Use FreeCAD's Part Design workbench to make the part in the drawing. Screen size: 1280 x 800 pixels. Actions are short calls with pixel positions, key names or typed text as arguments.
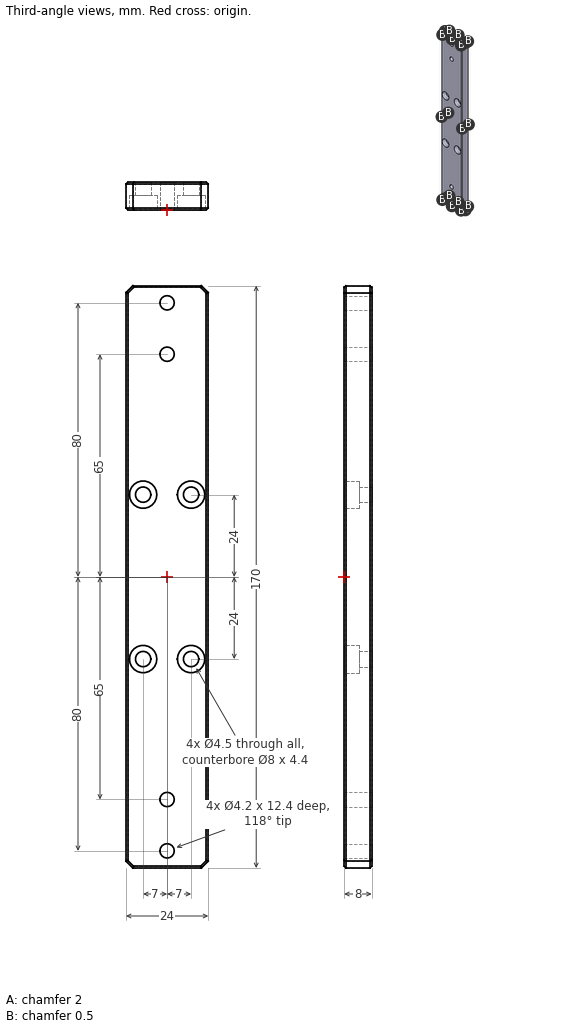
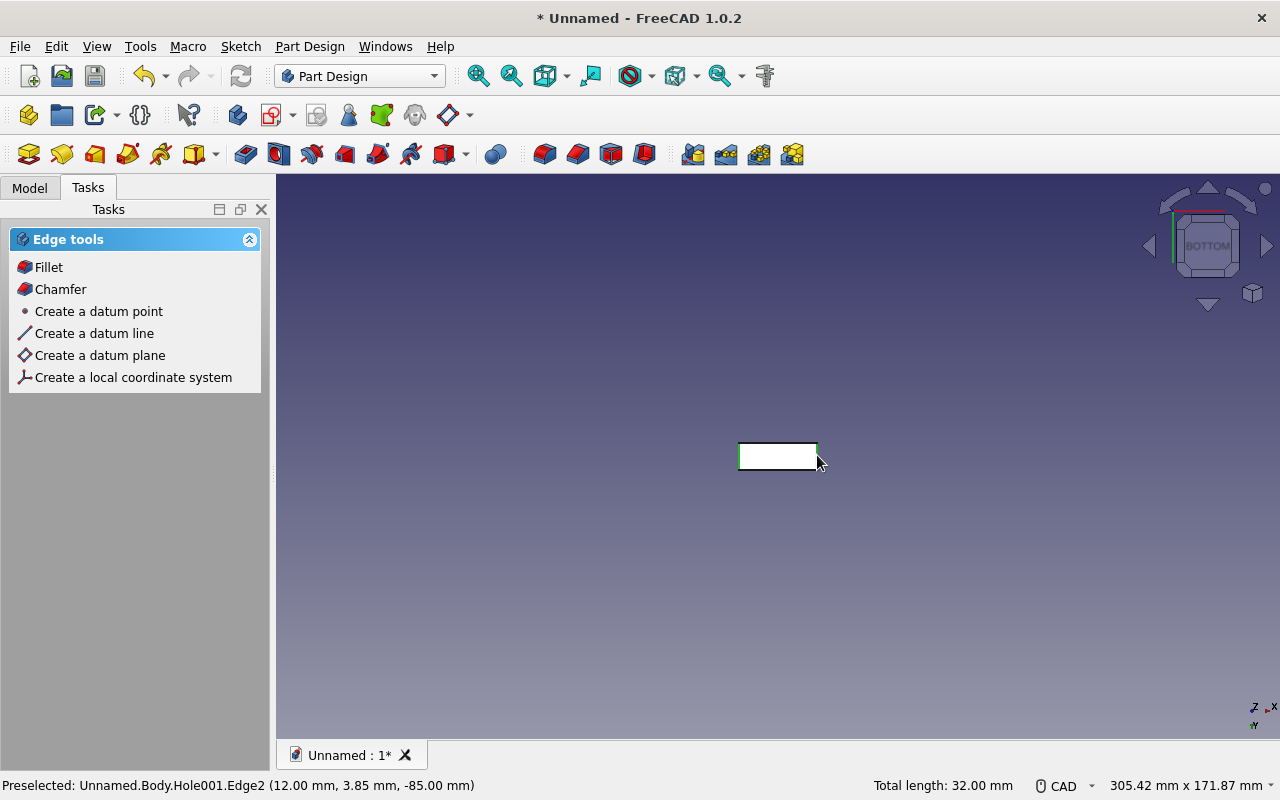
click(578, 154)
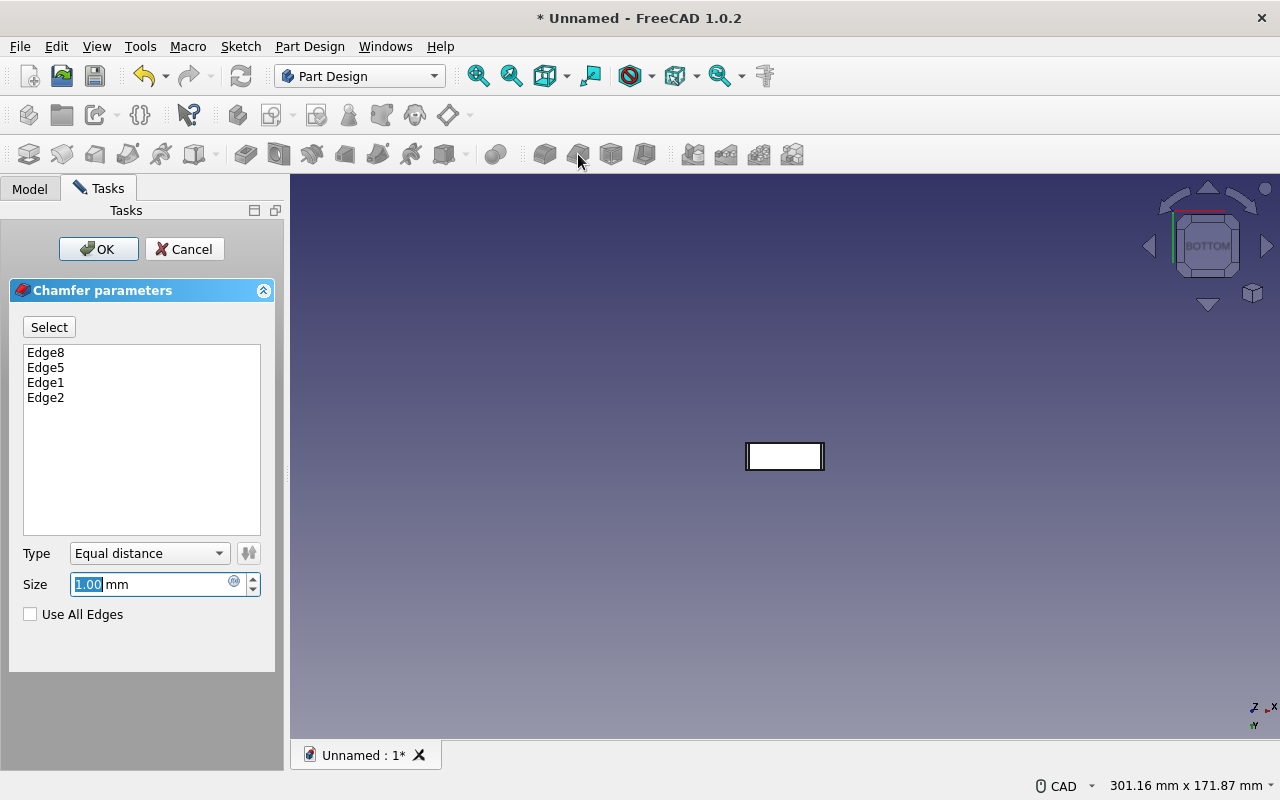
text(2)
key(Tab)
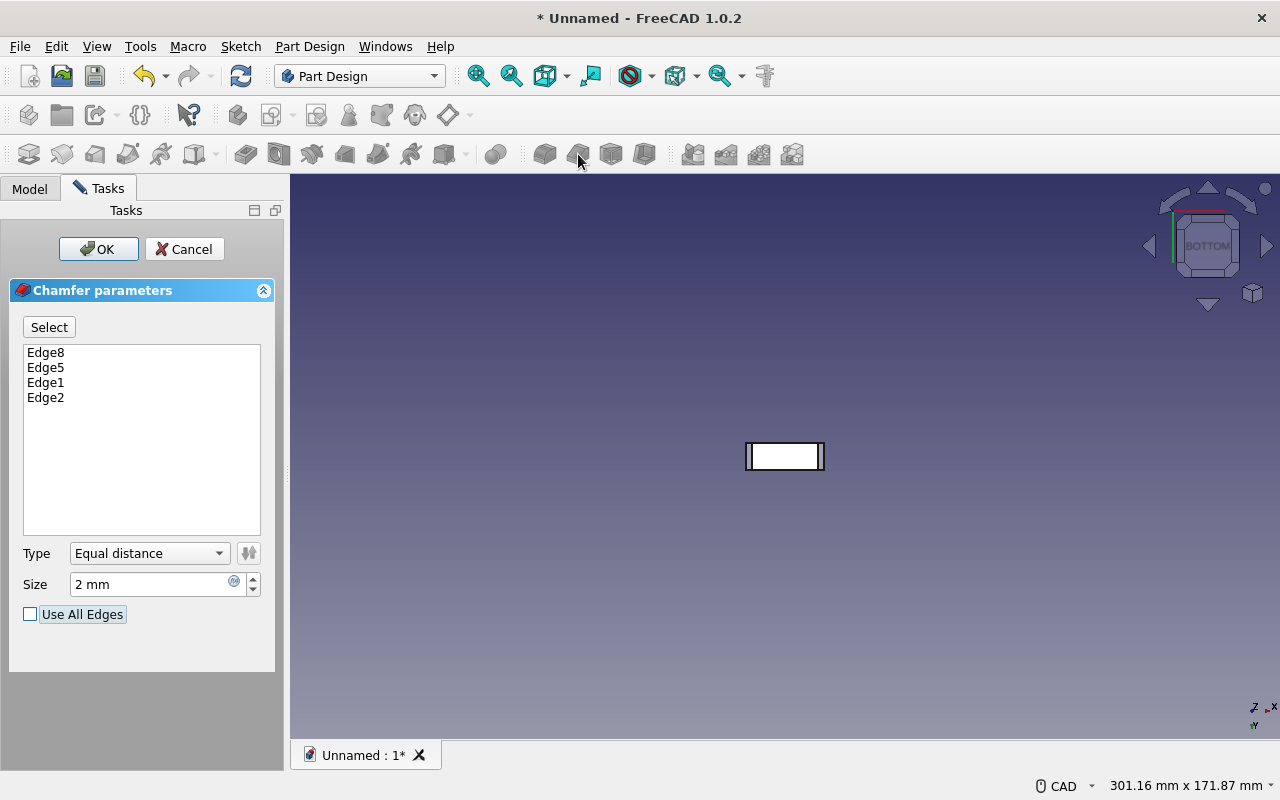
click(99, 249)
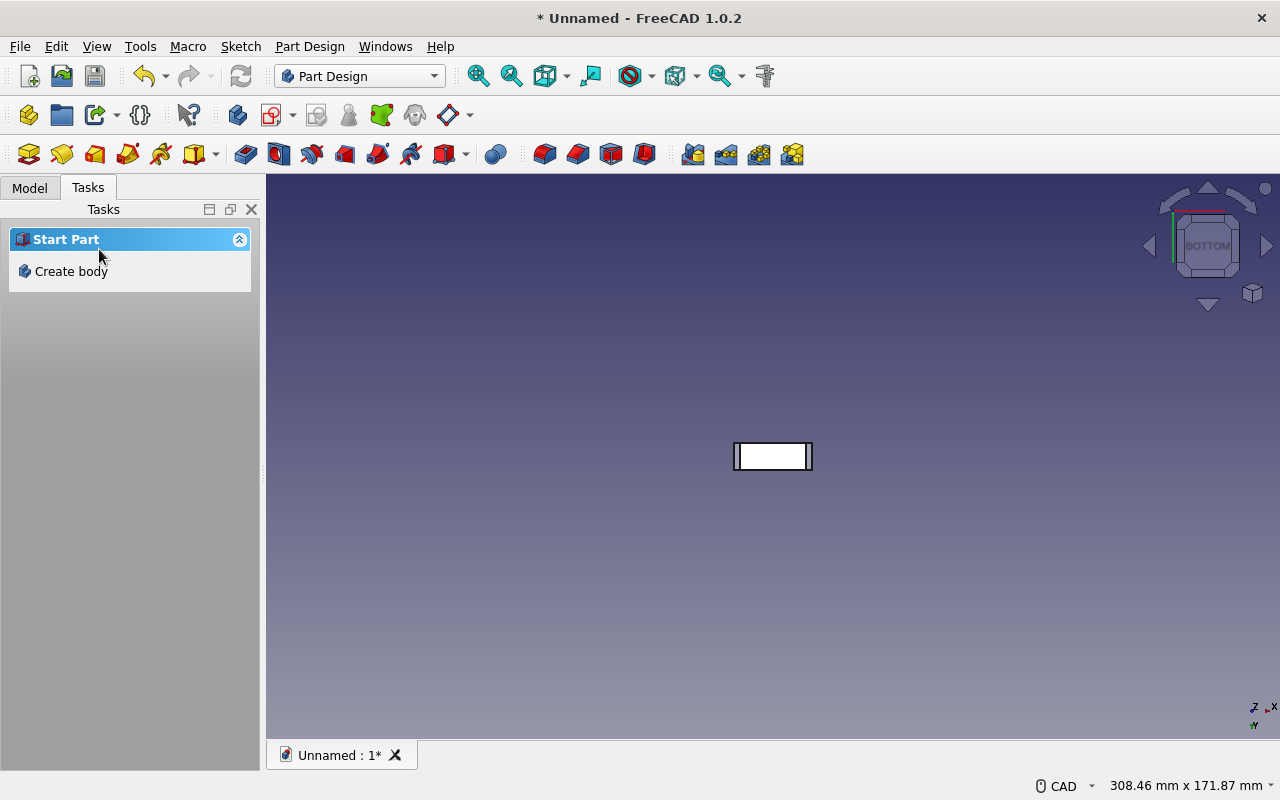
click(479, 76)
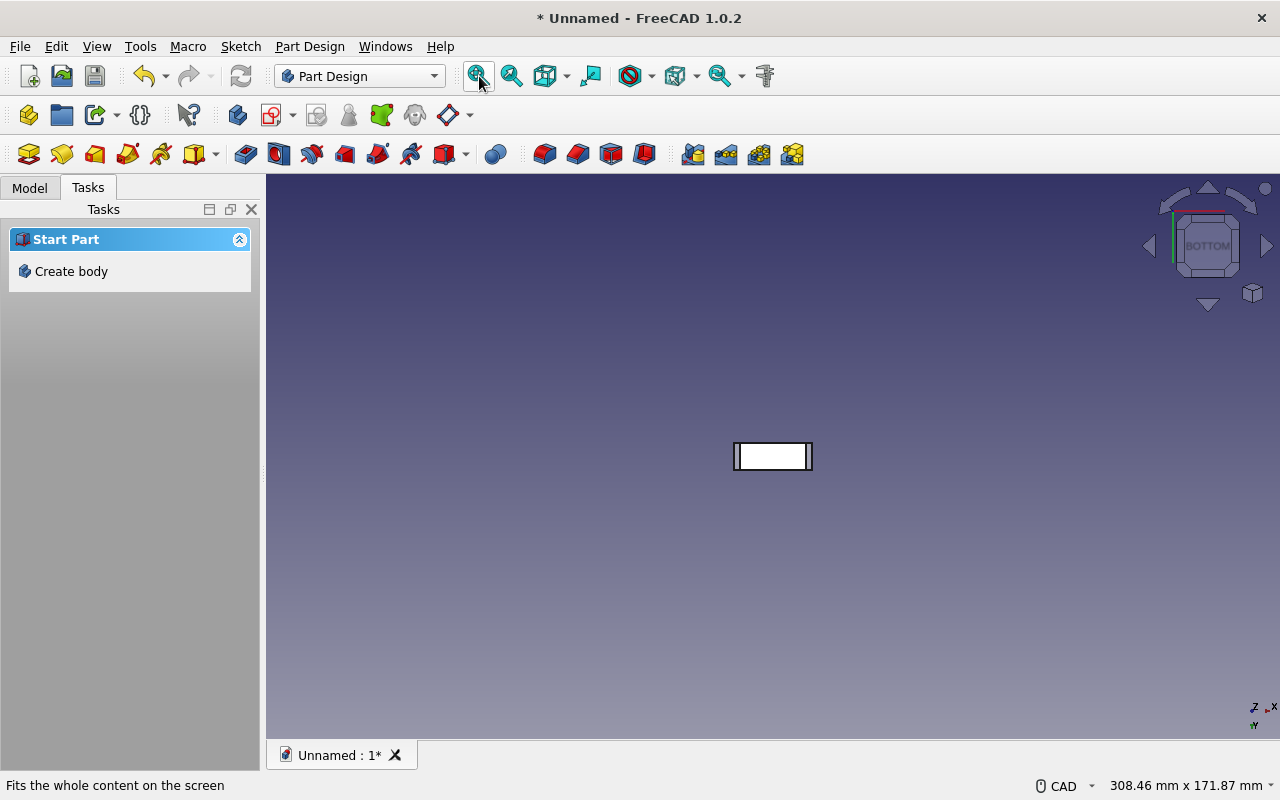
click(773, 442)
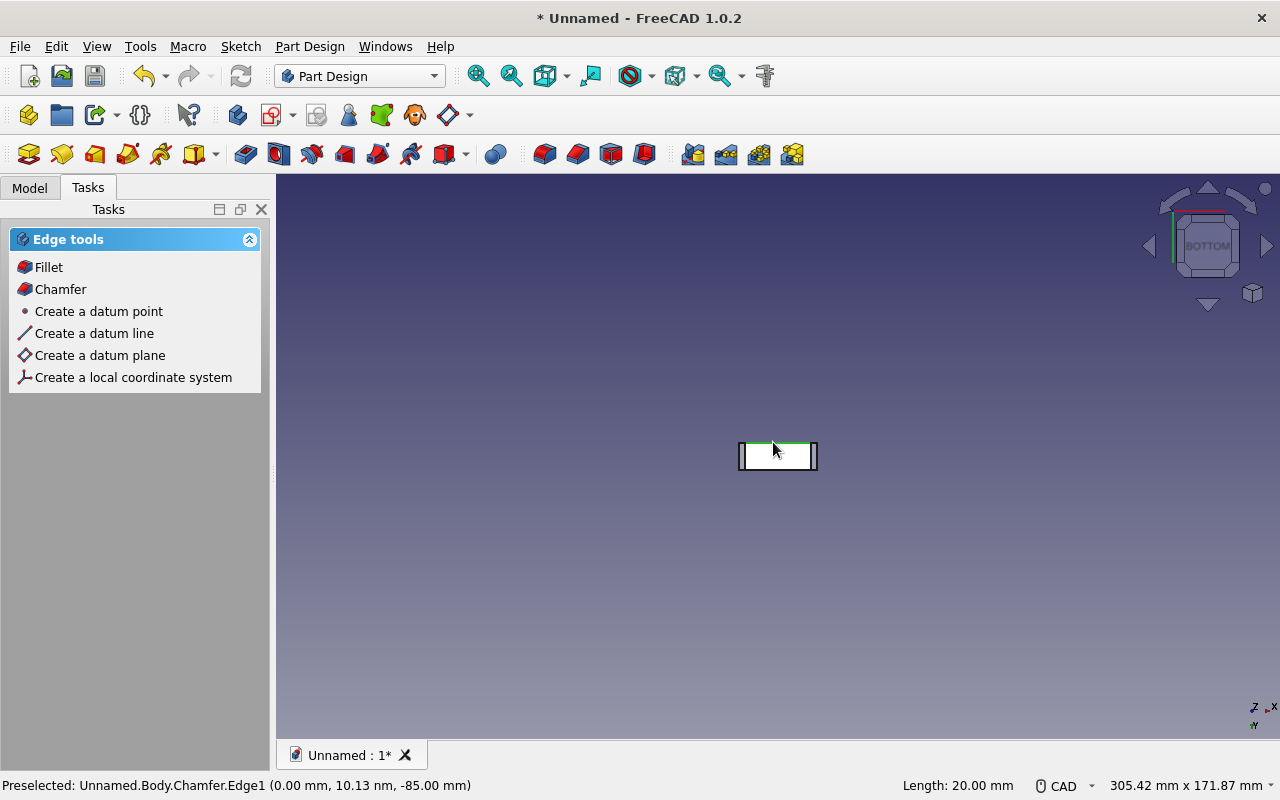
key(0)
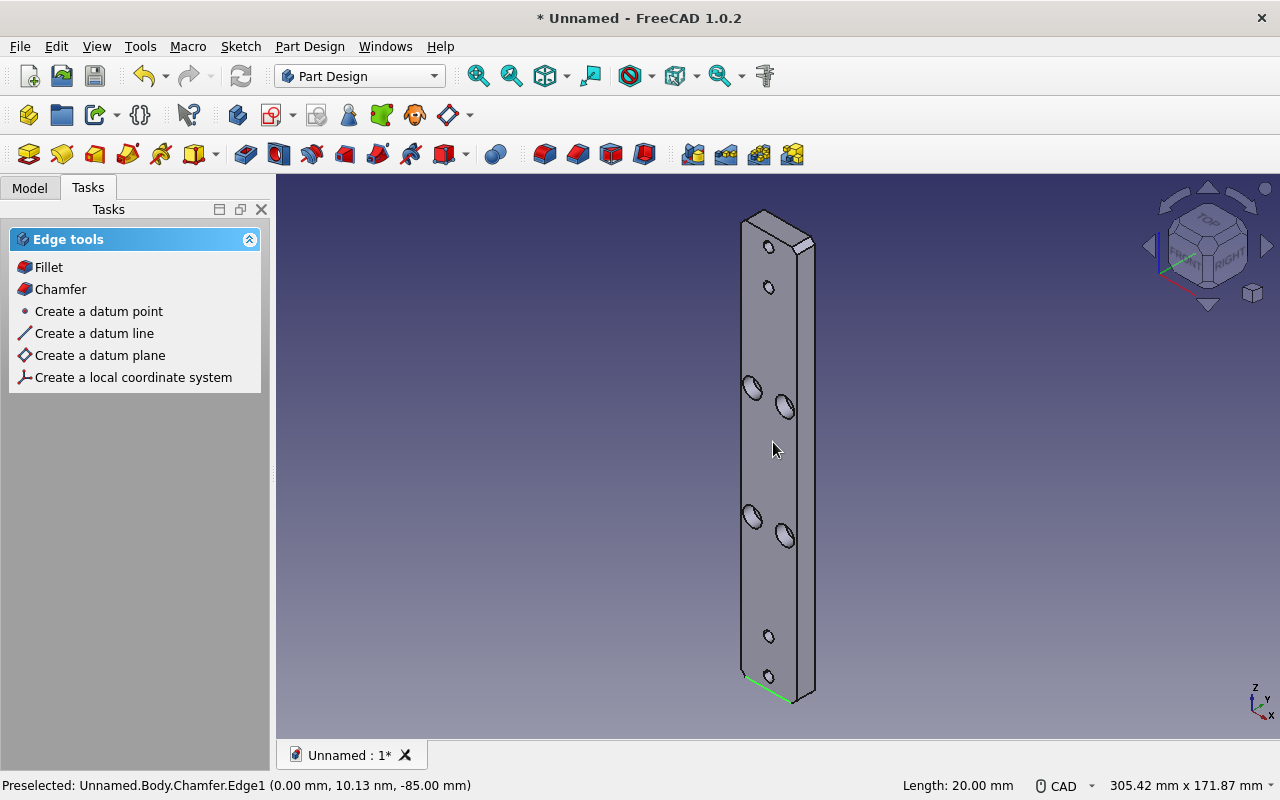
click(797, 477, ctrl)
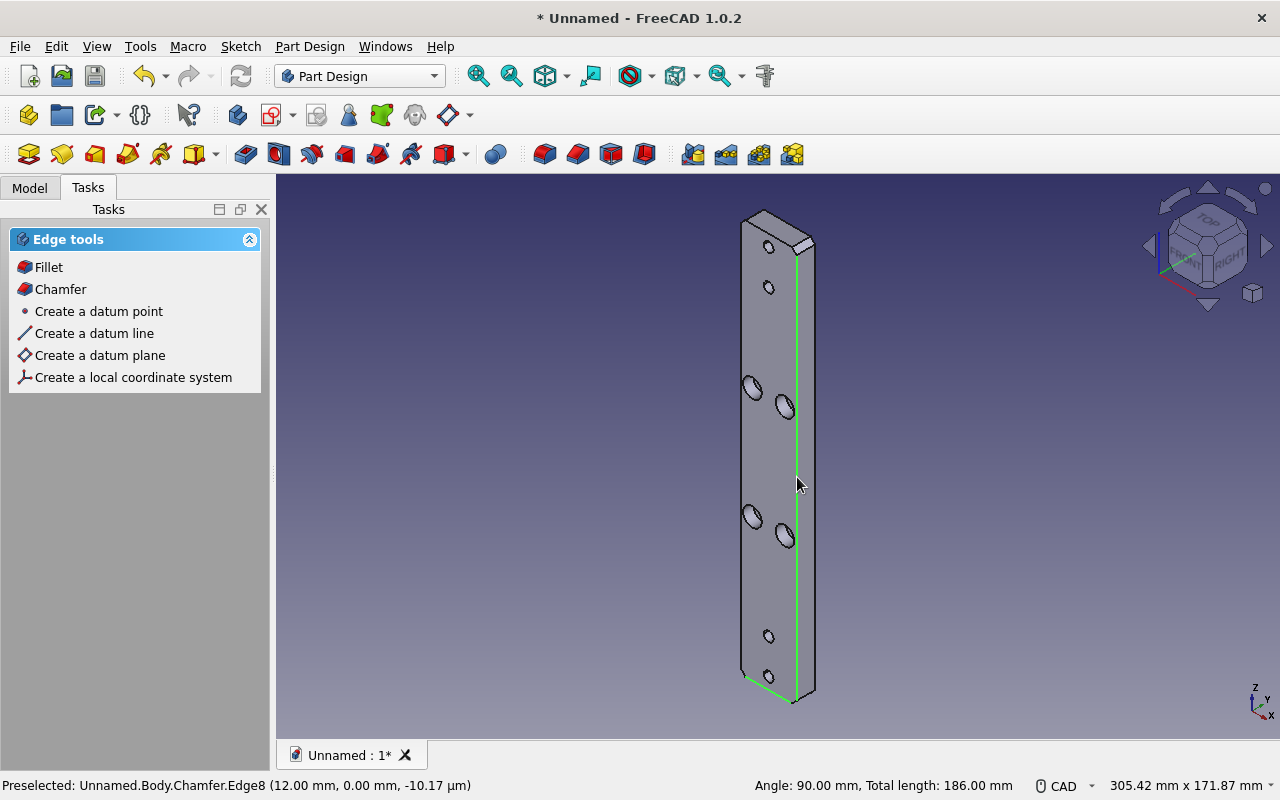
click(769, 233, ctrl)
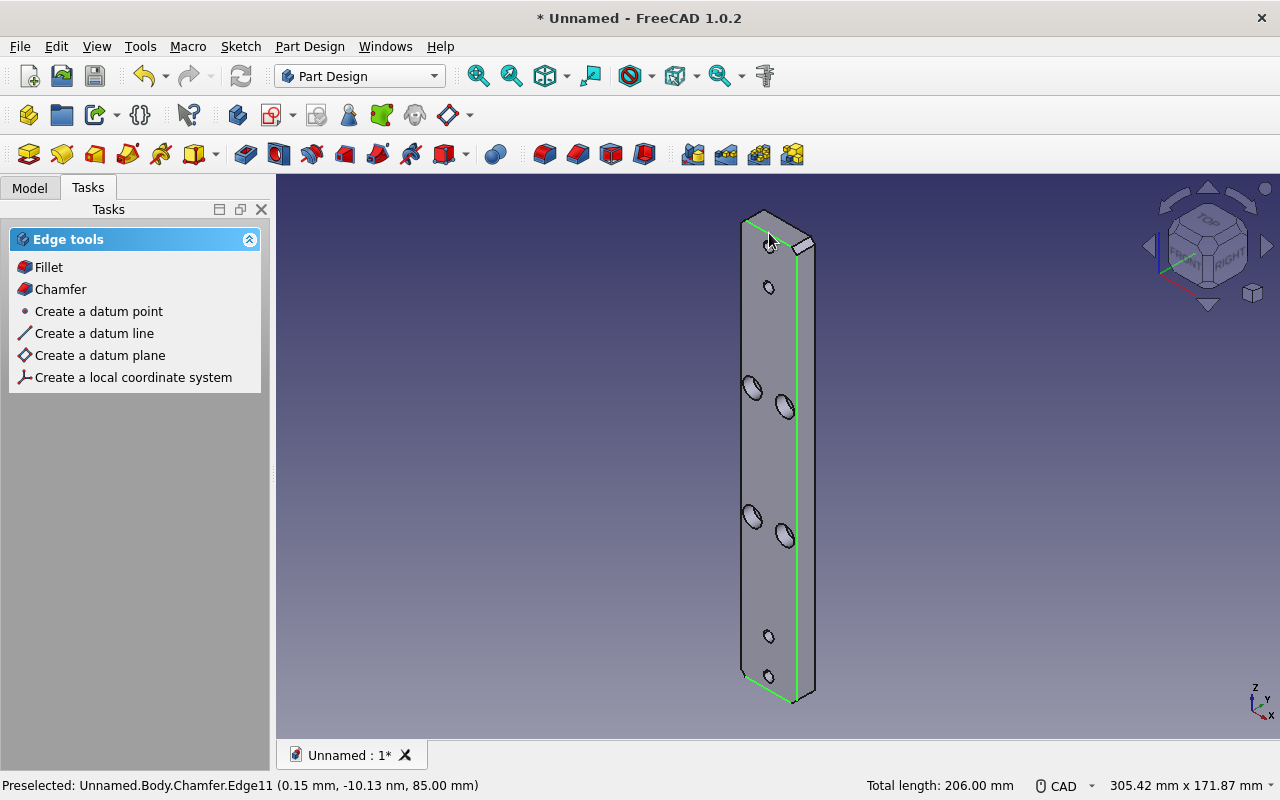
key(2)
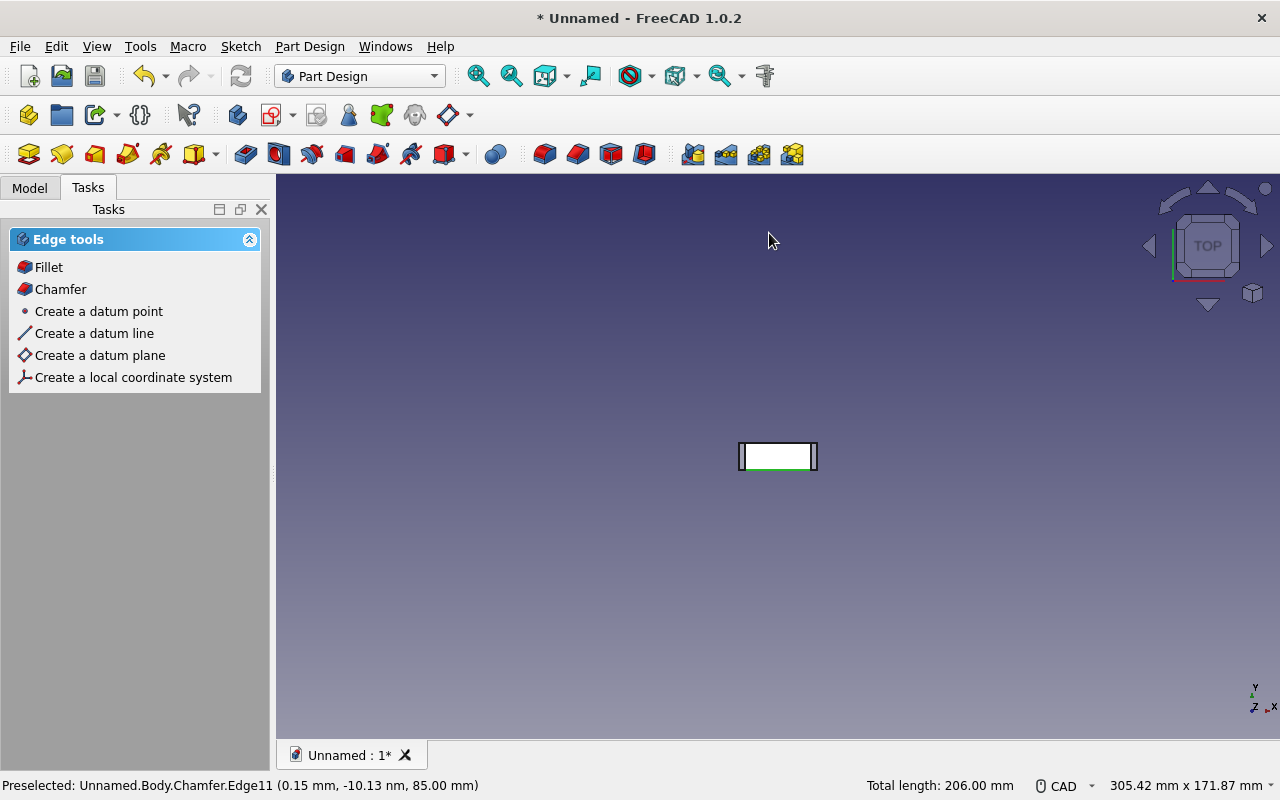
click(479, 76)